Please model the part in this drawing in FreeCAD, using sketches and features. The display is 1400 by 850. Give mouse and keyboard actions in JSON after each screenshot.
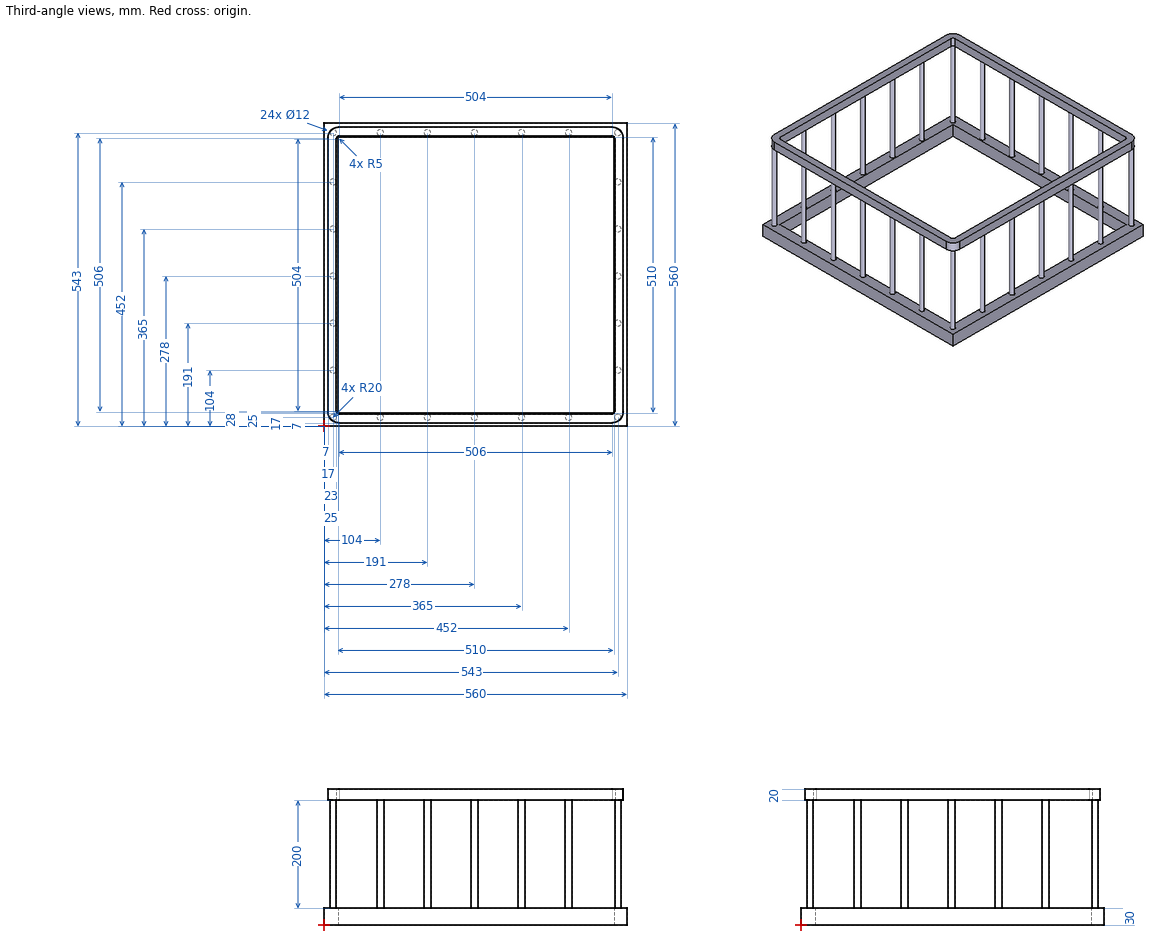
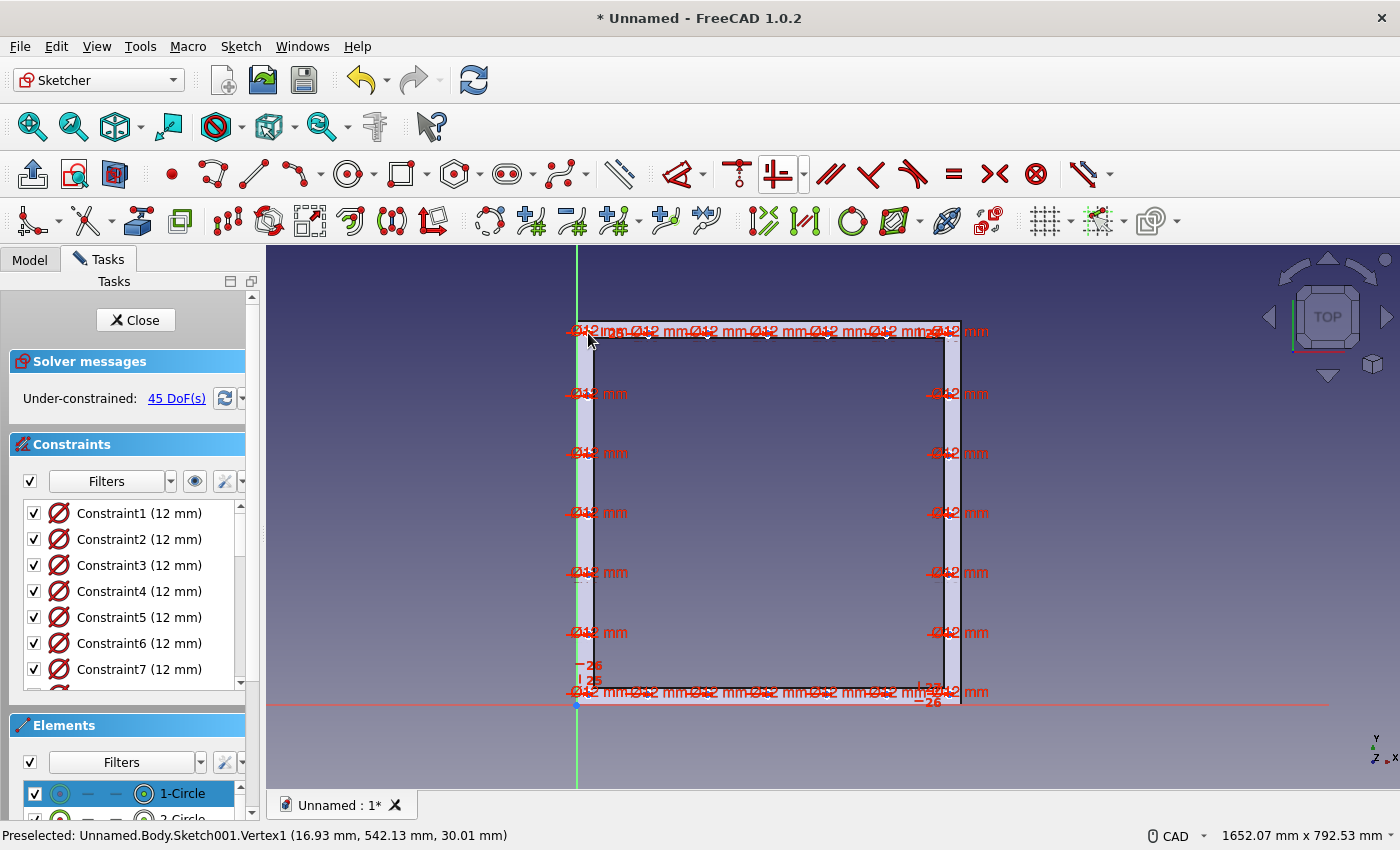
{"action": "left_click", "coordinate": [949, 334]}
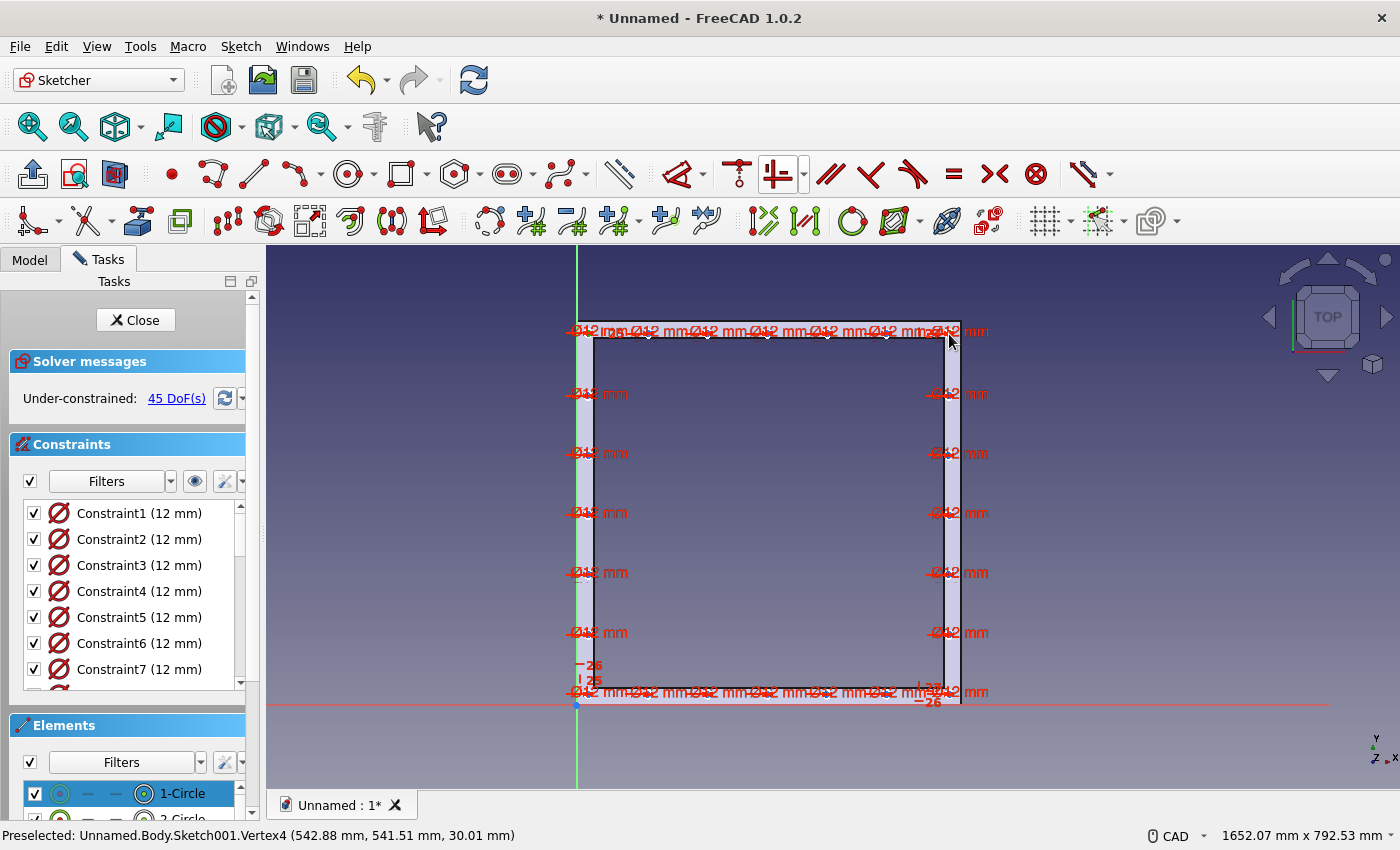
{"action": "key", "text": "h"}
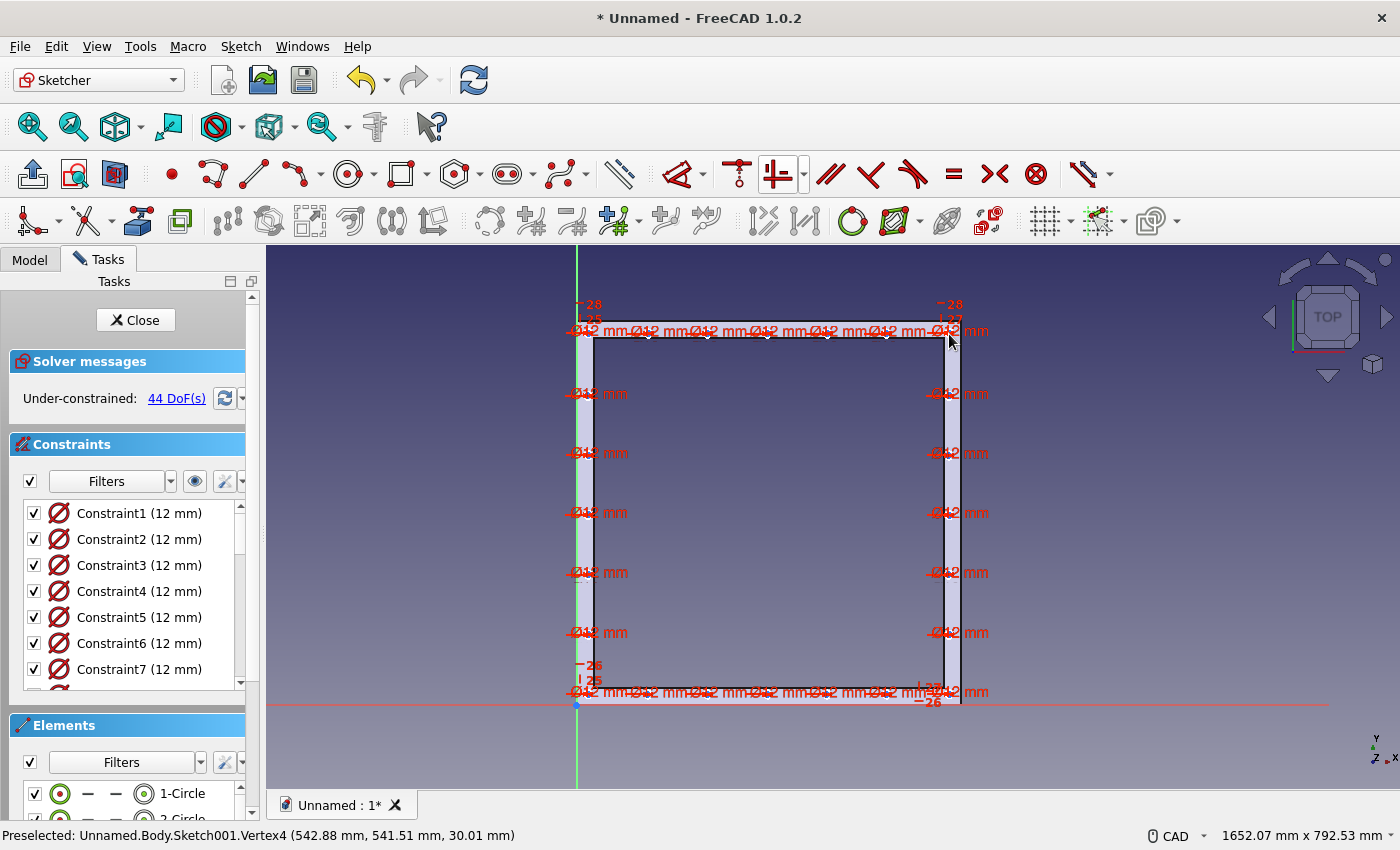
{"action": "left_click", "coordinate": [588, 333]}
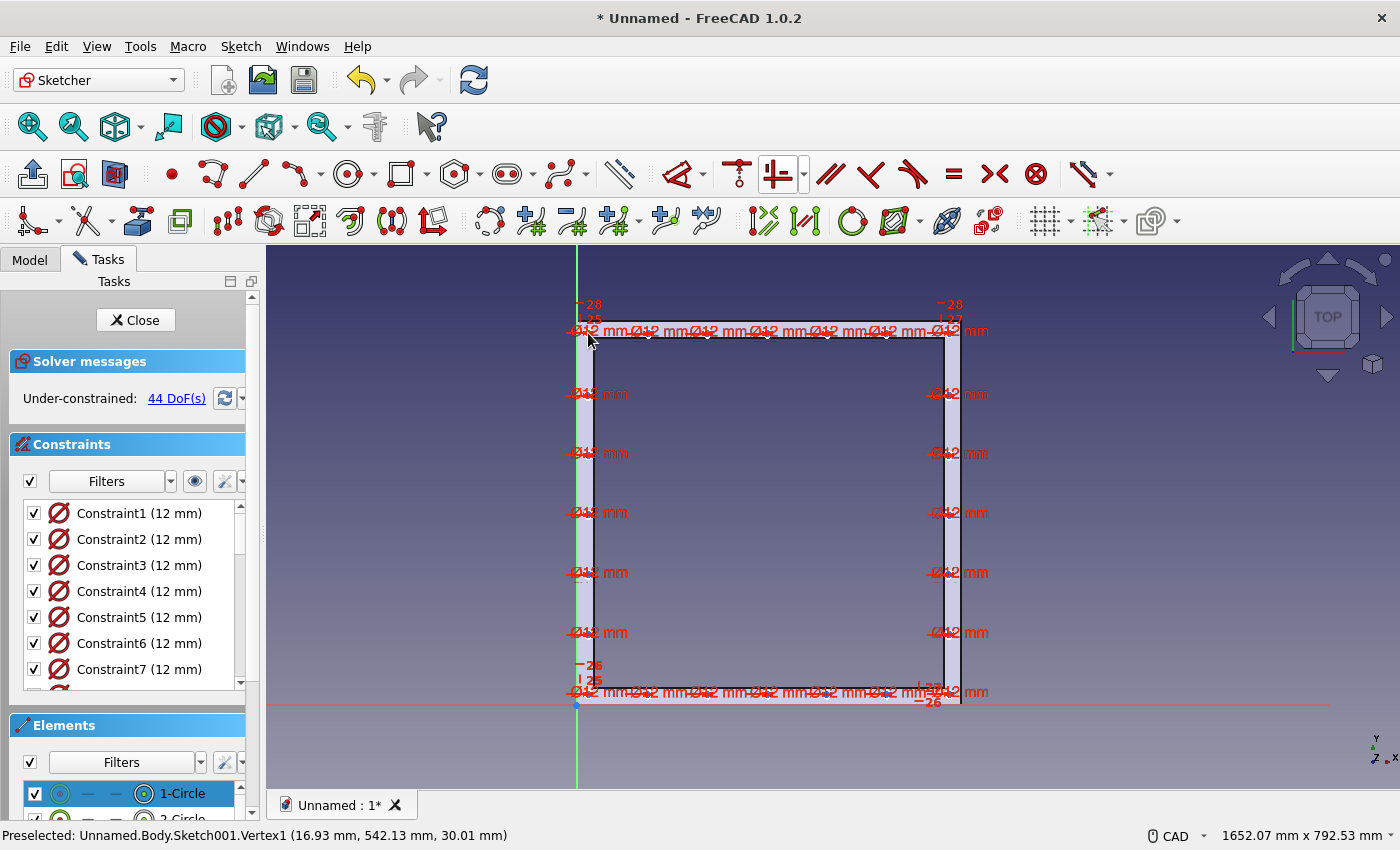
{"action": "left_click", "coordinate": [648, 334]}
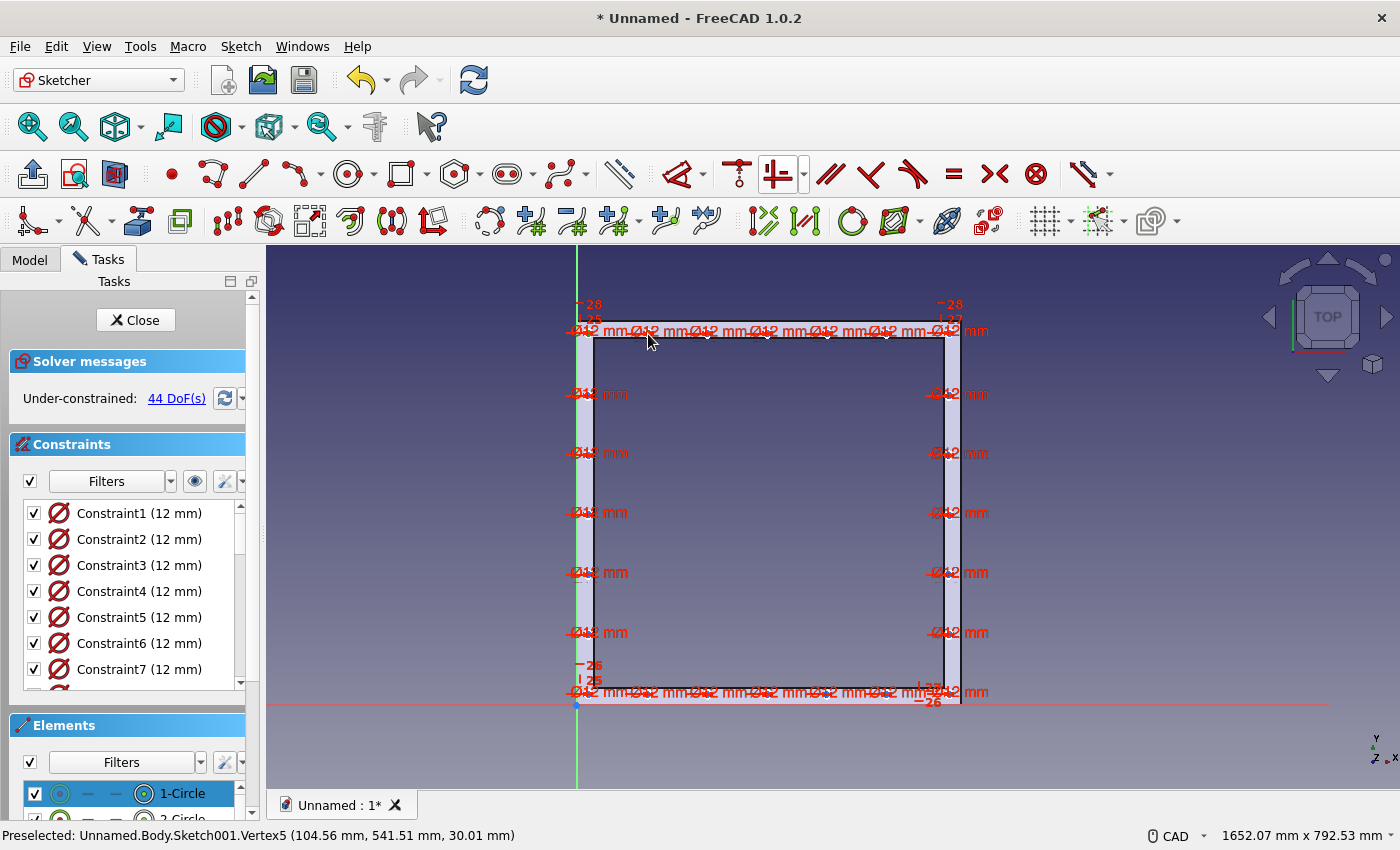
{"action": "left_click", "coordinate": [804, 174]}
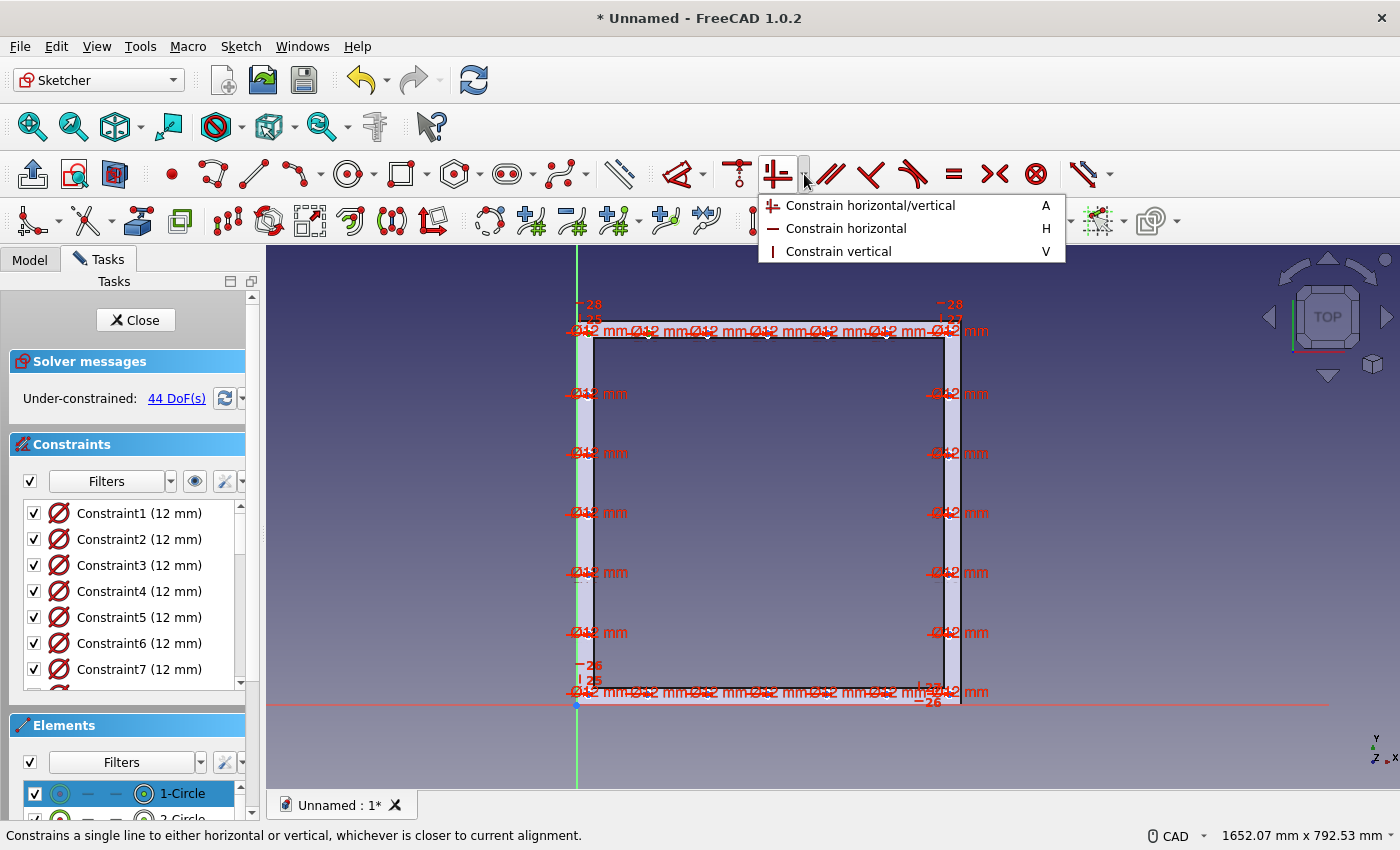
{"action": "left_click", "coordinate": [912, 228]}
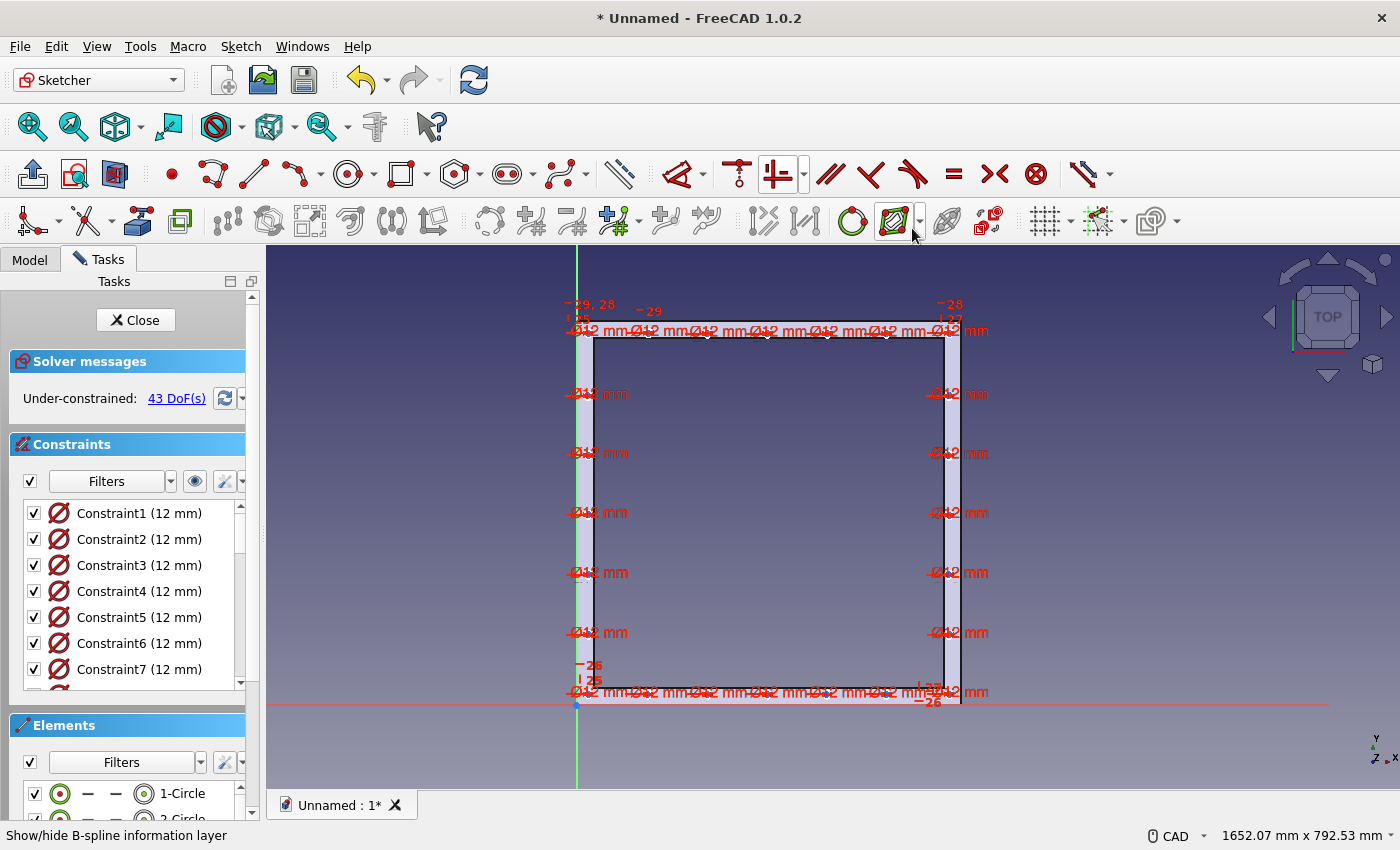
{"action": "left_click", "coordinate": [648, 333]}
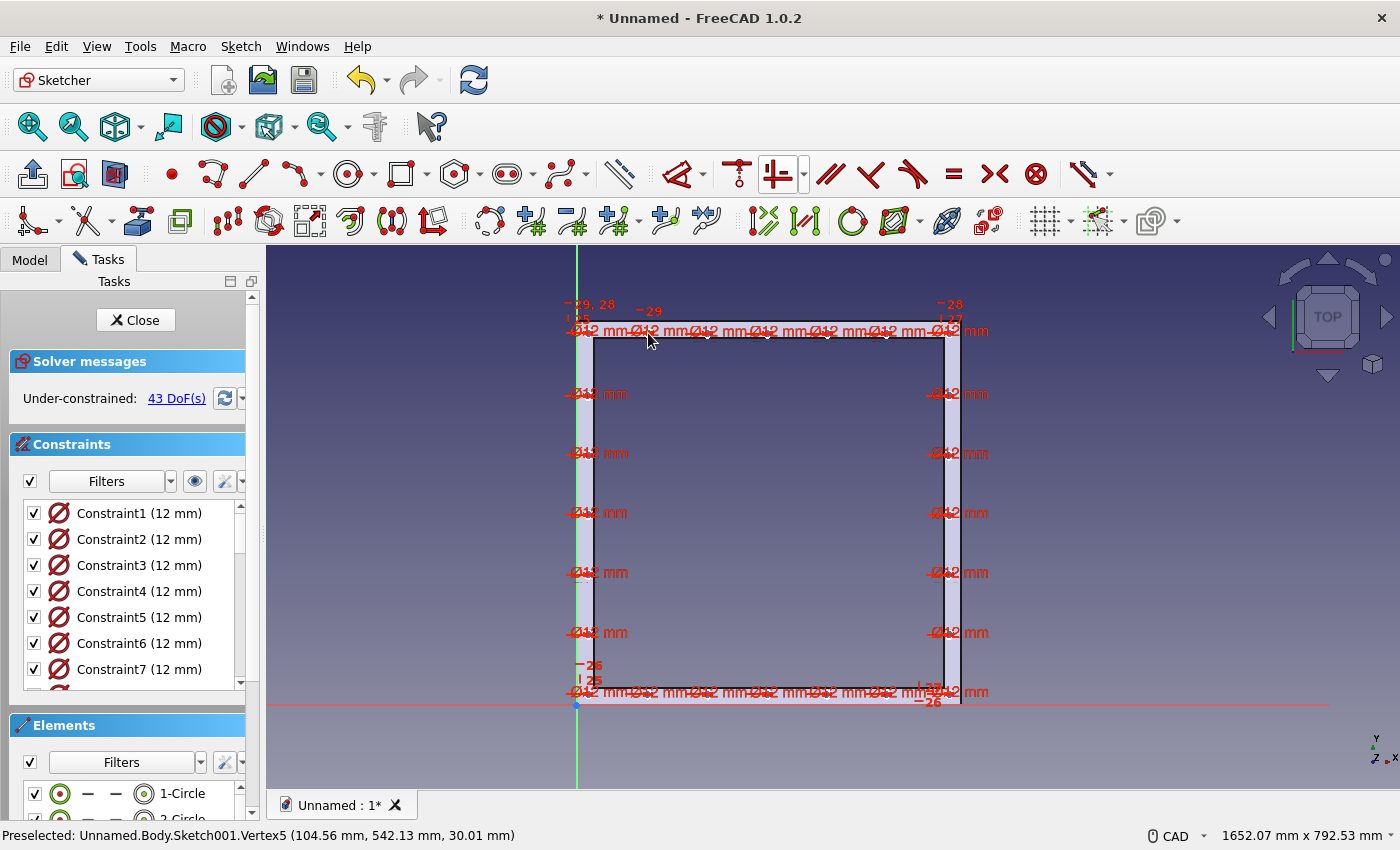
{"action": "left_click", "coordinate": [648, 694]}